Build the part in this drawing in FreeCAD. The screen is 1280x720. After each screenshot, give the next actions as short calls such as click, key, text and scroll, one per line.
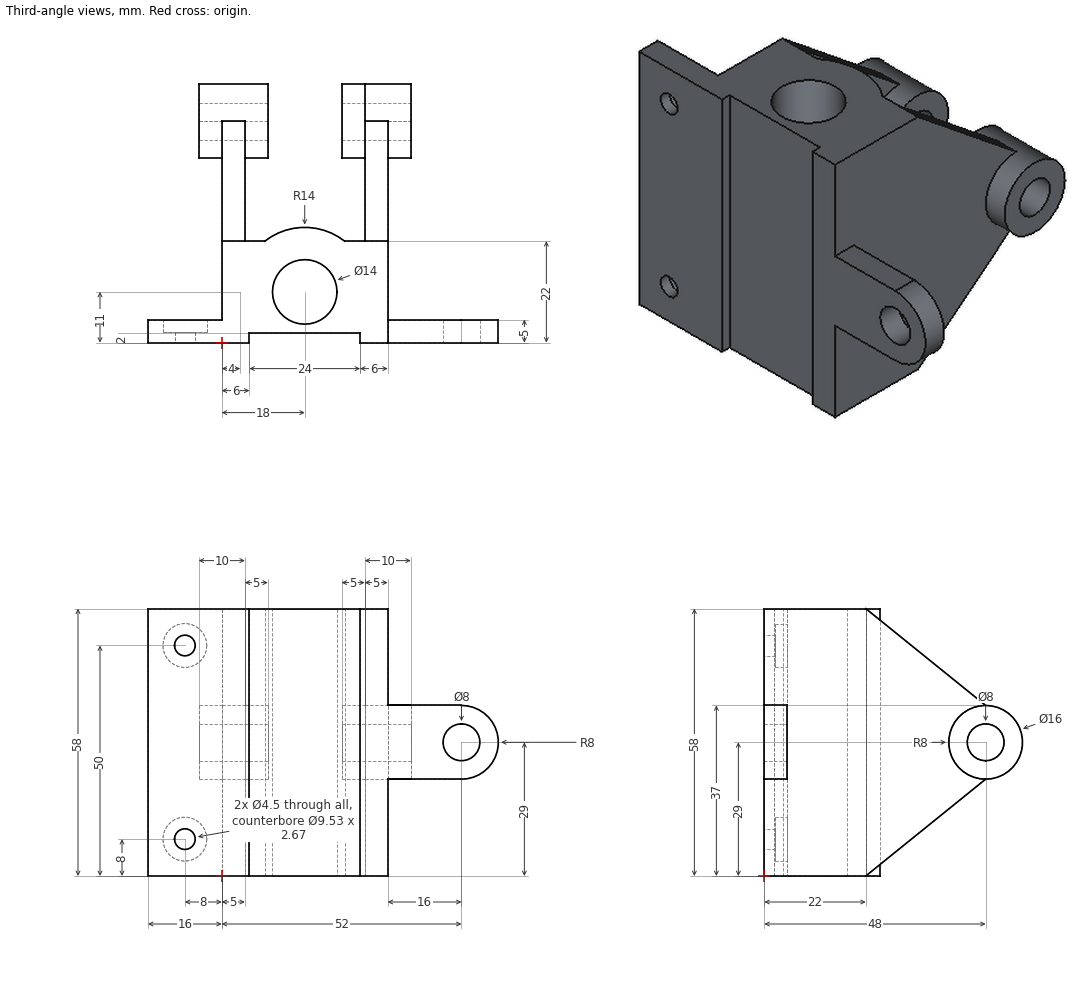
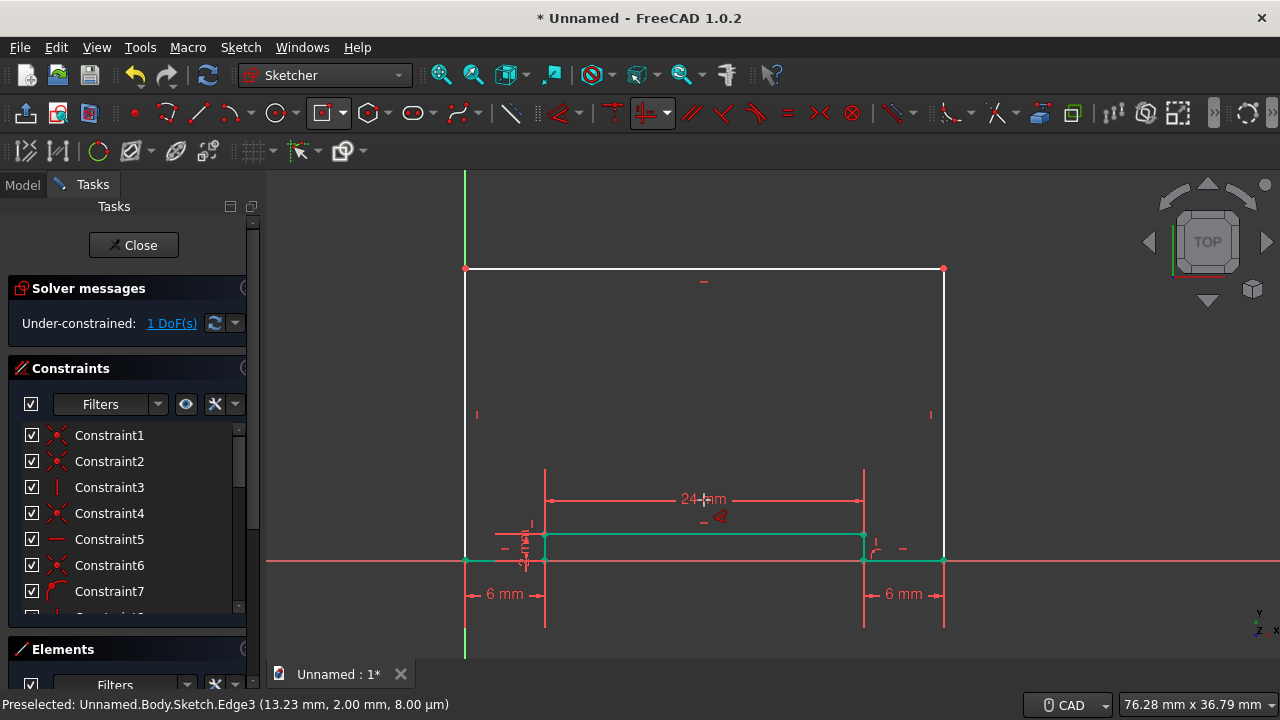
click(944, 473)
click(978, 415)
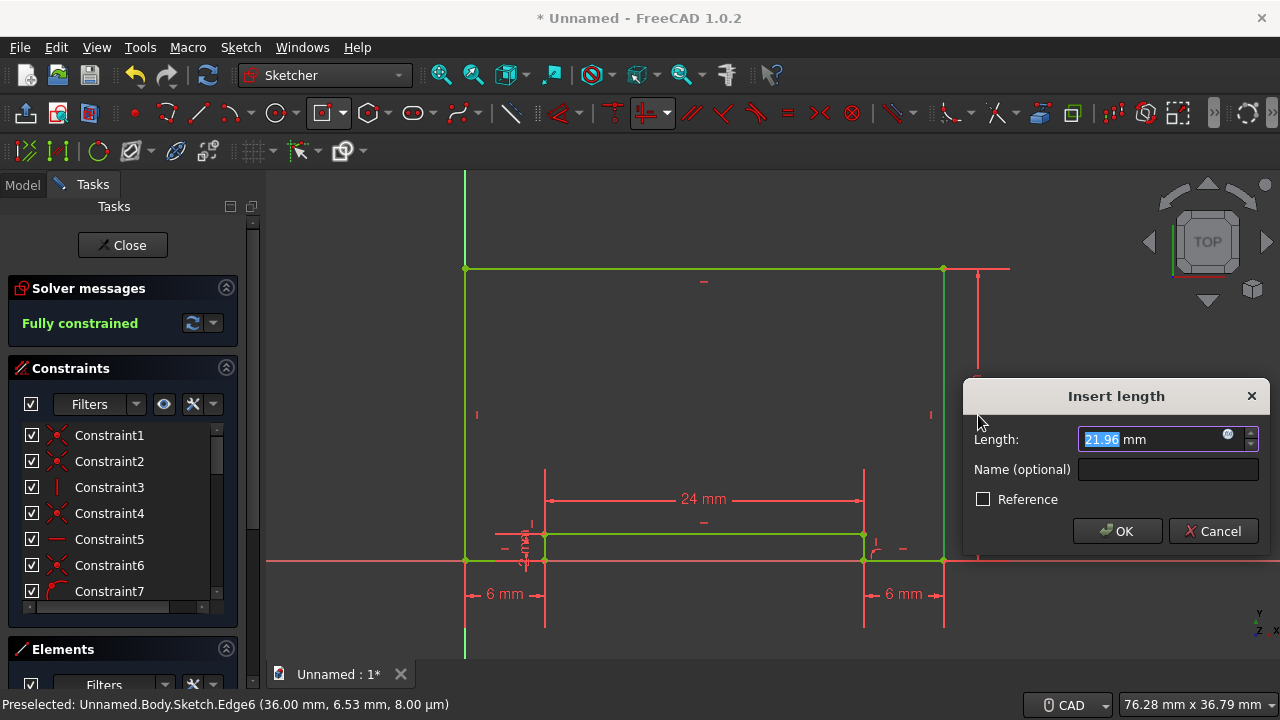
text(22)
key(Return)
key(Escape)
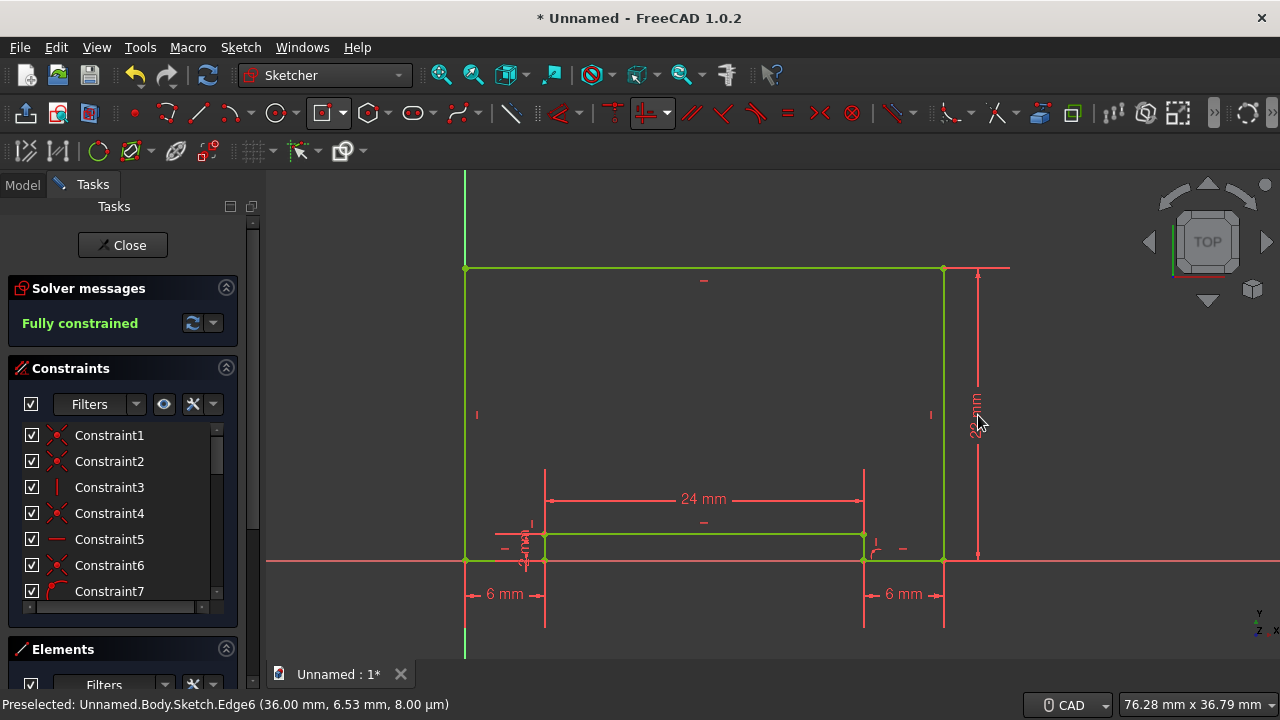
click(123, 245)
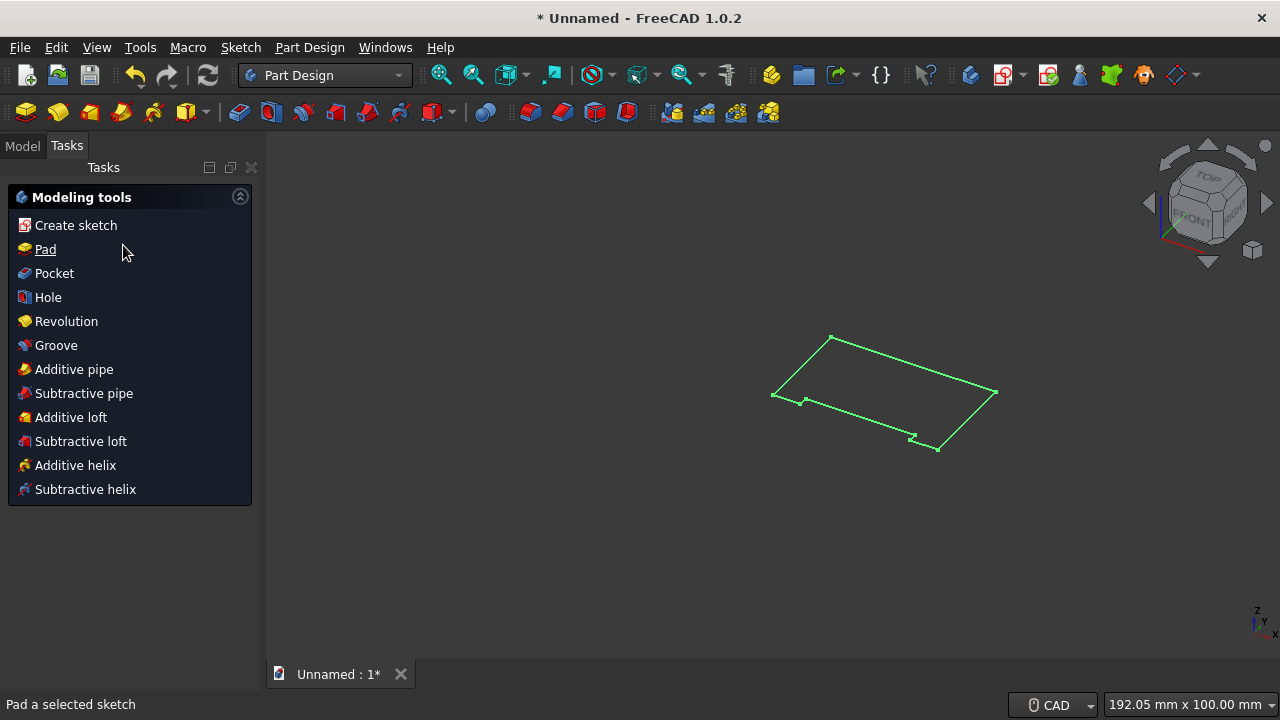
click(26, 112)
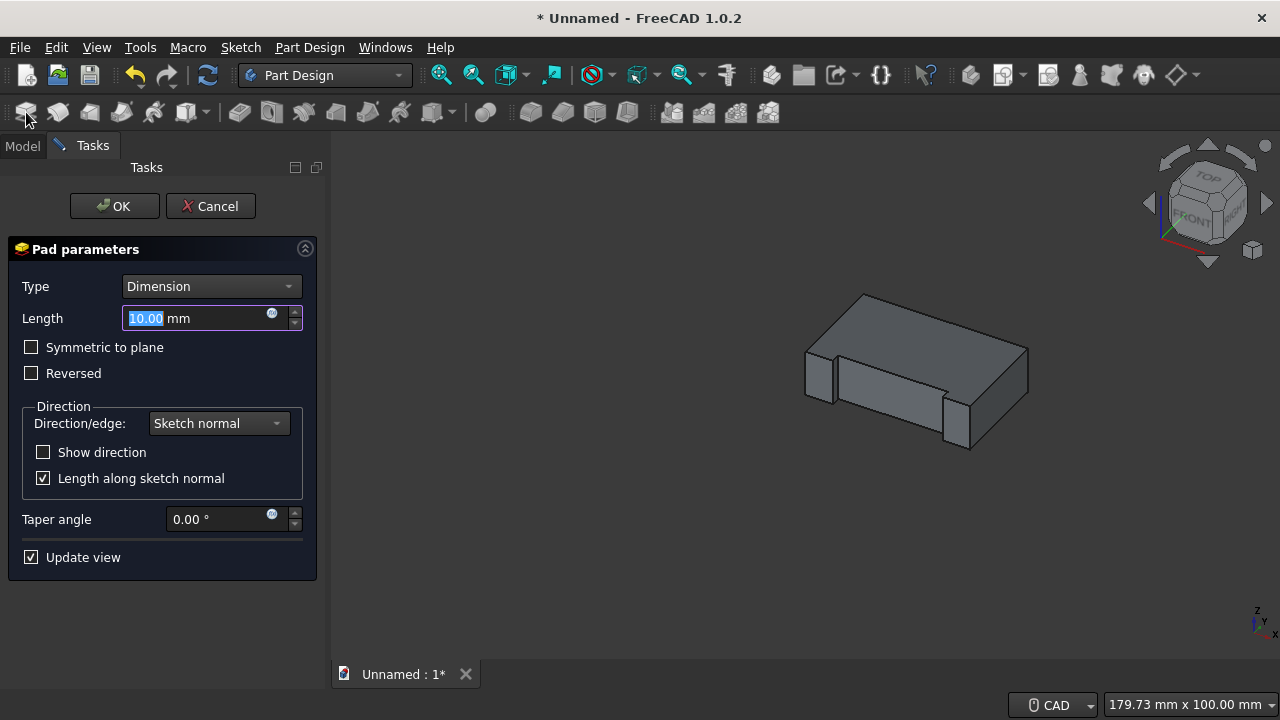
text(58)
key(Tab)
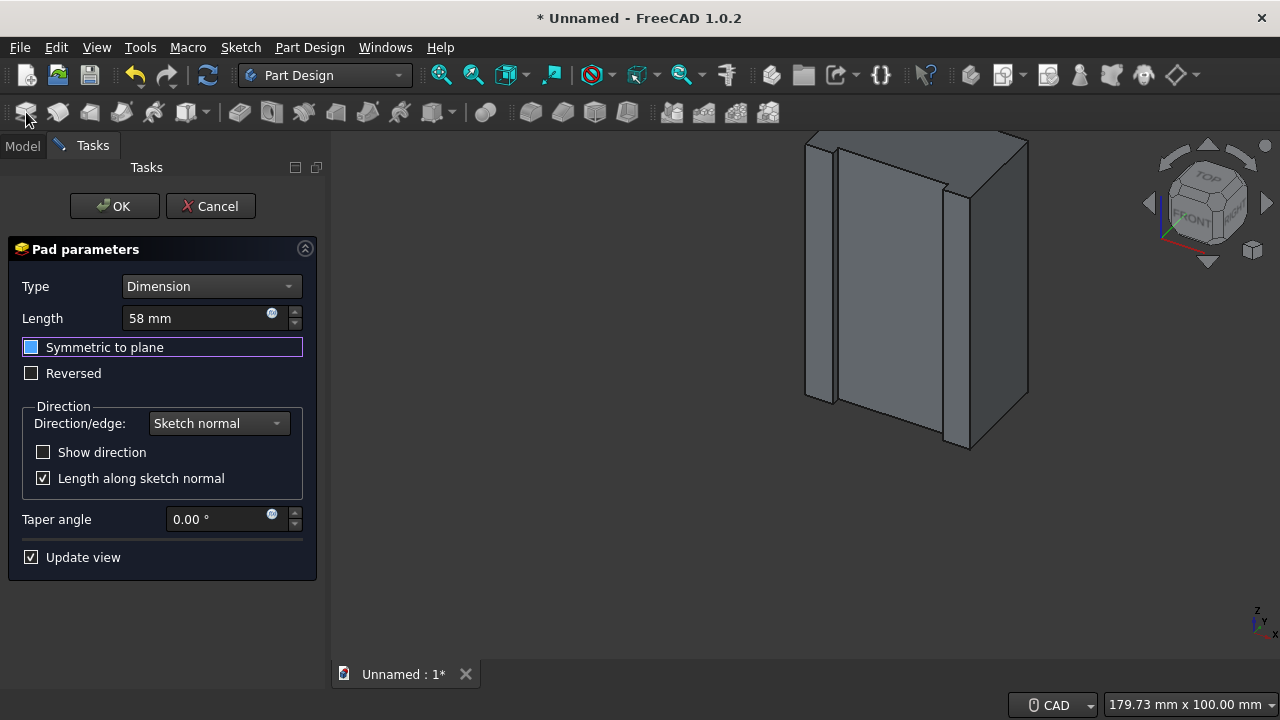
click(115, 206)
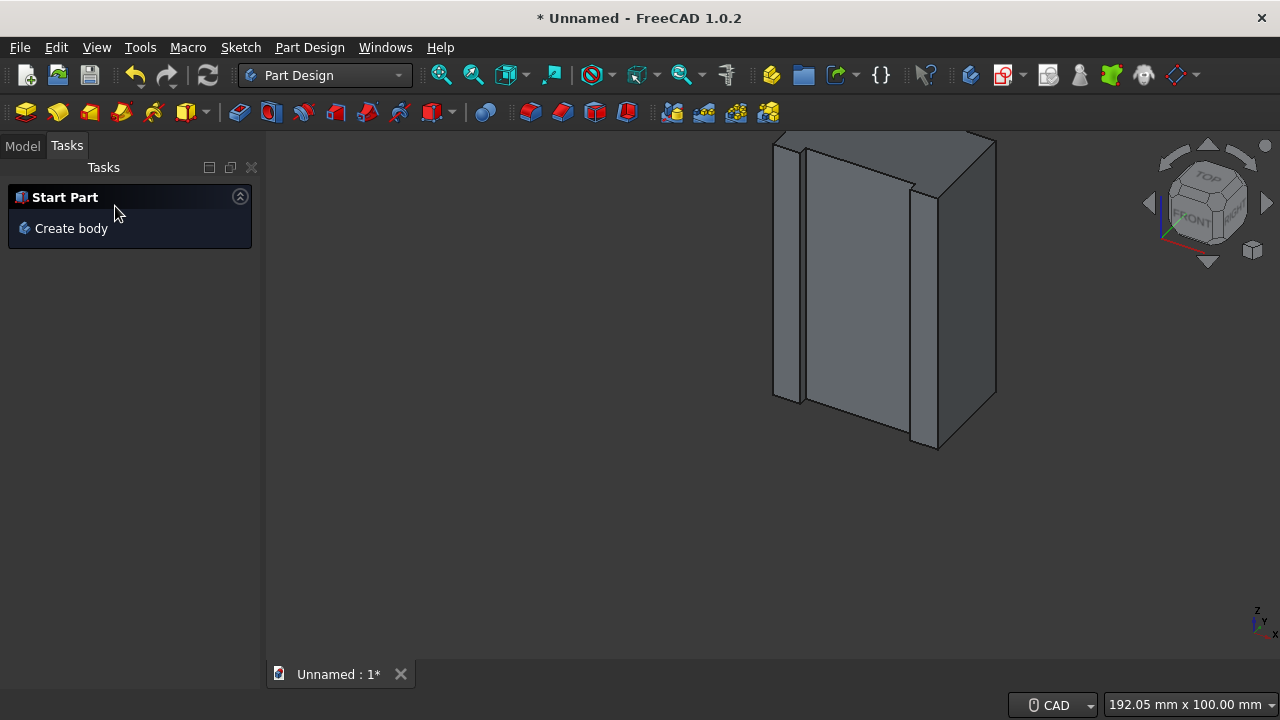
key(v)
key(f)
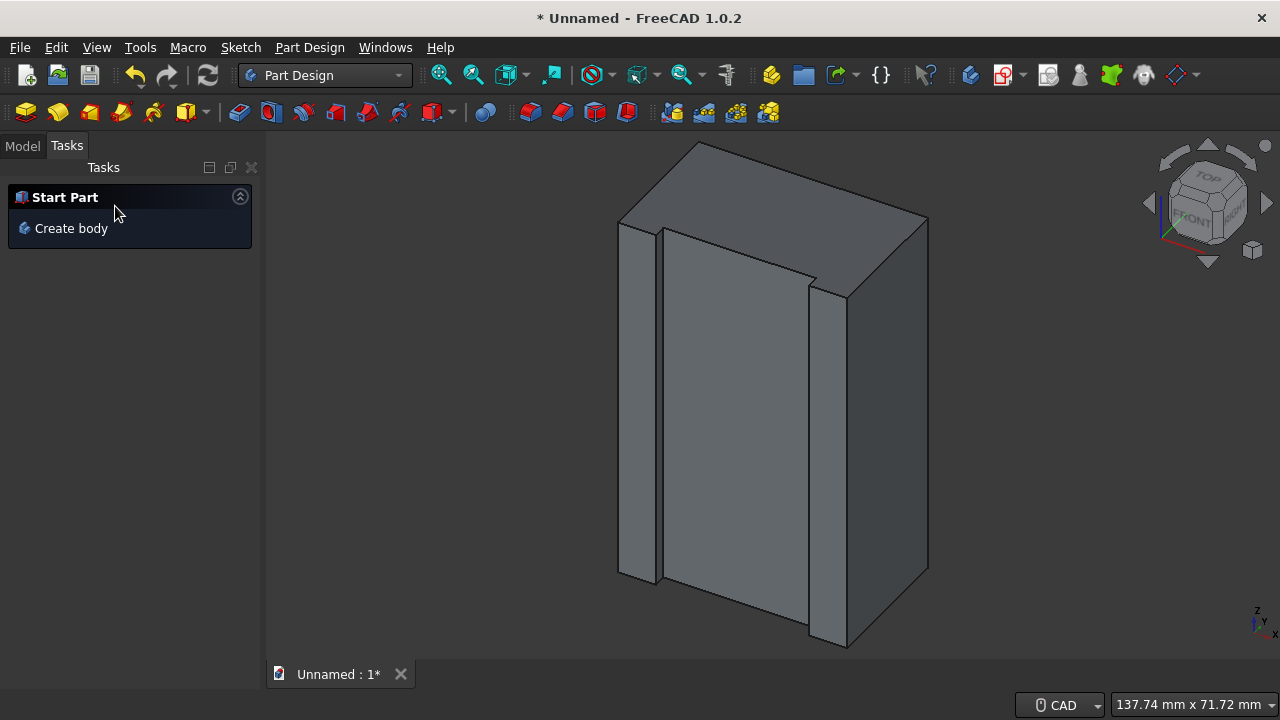
click(806, 230)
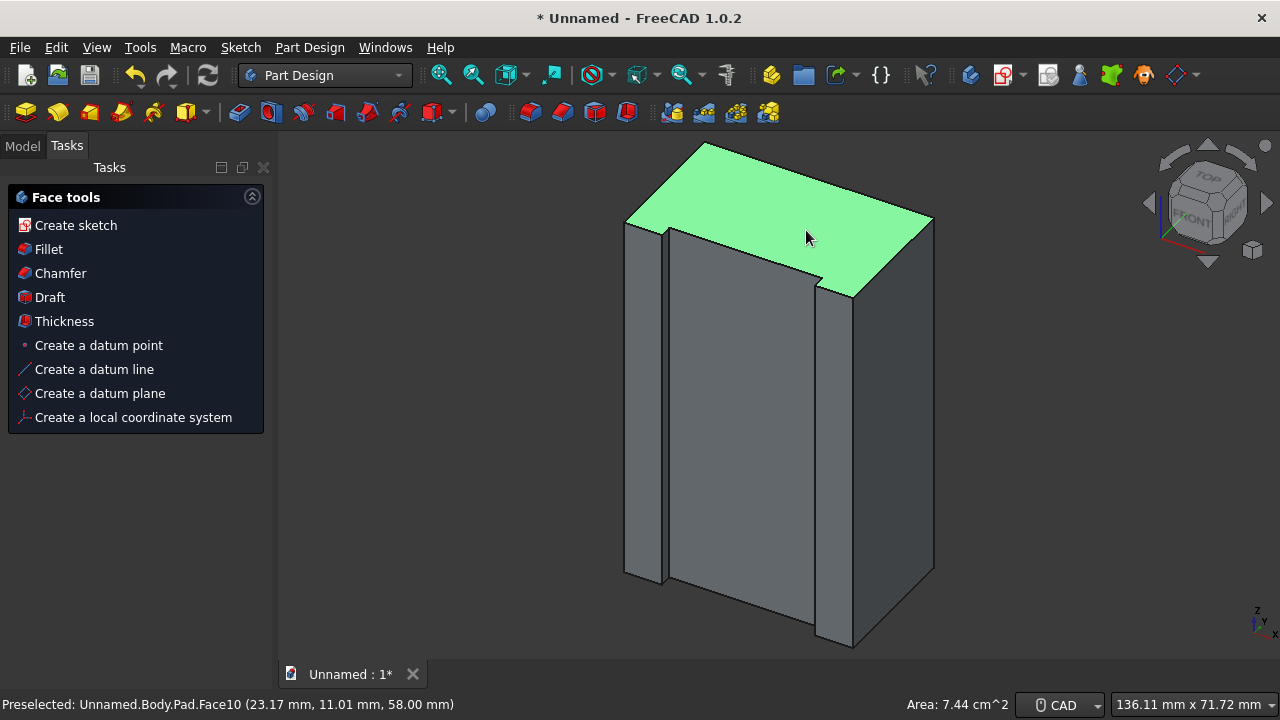
click(1004, 76)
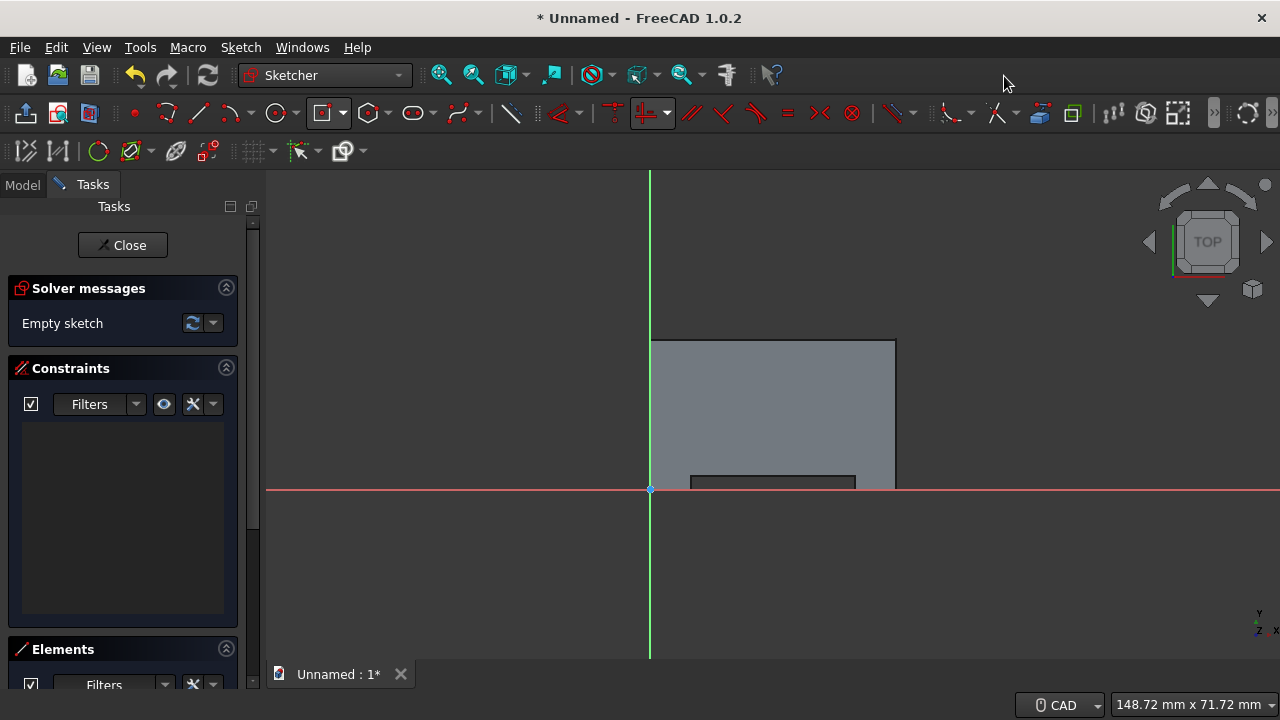
scroll(826, 392, up, 3)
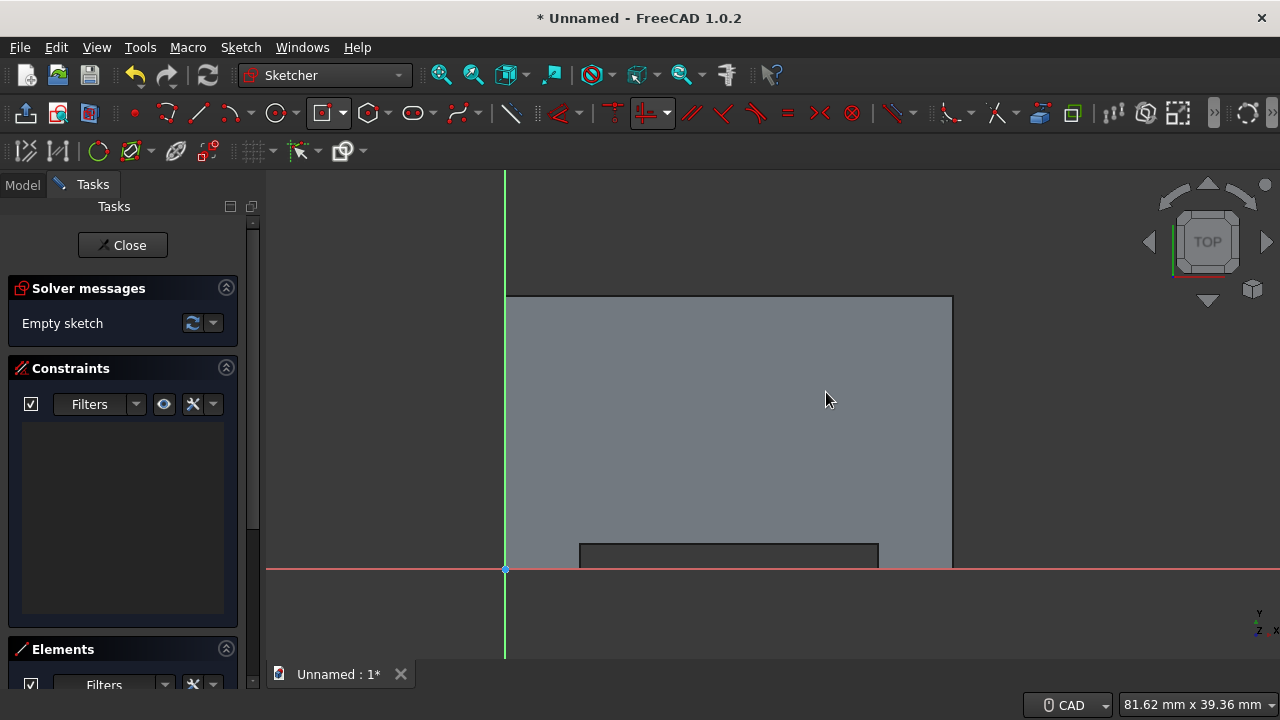
key(g)
key(l)